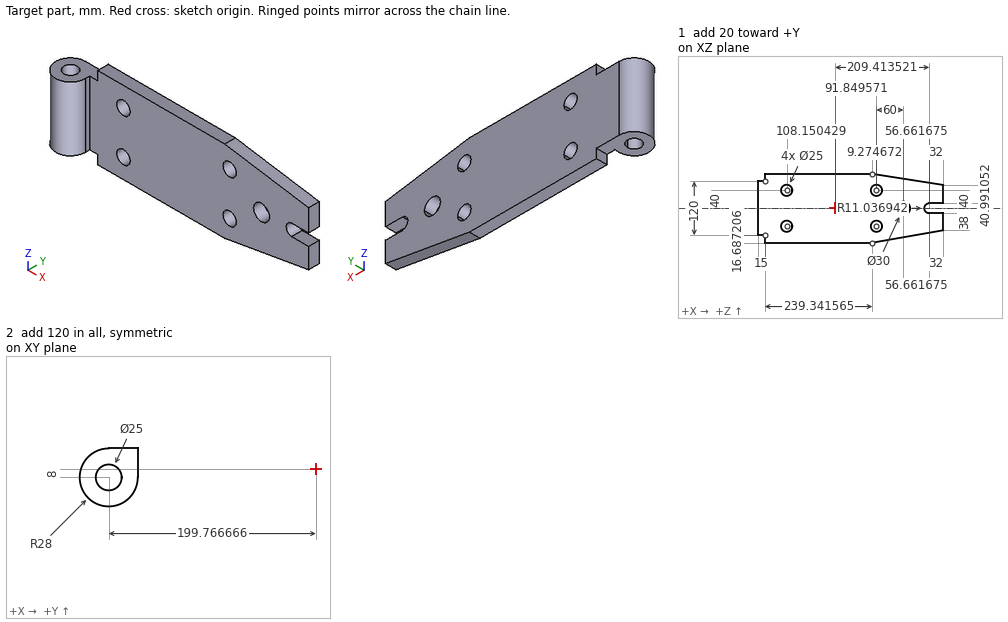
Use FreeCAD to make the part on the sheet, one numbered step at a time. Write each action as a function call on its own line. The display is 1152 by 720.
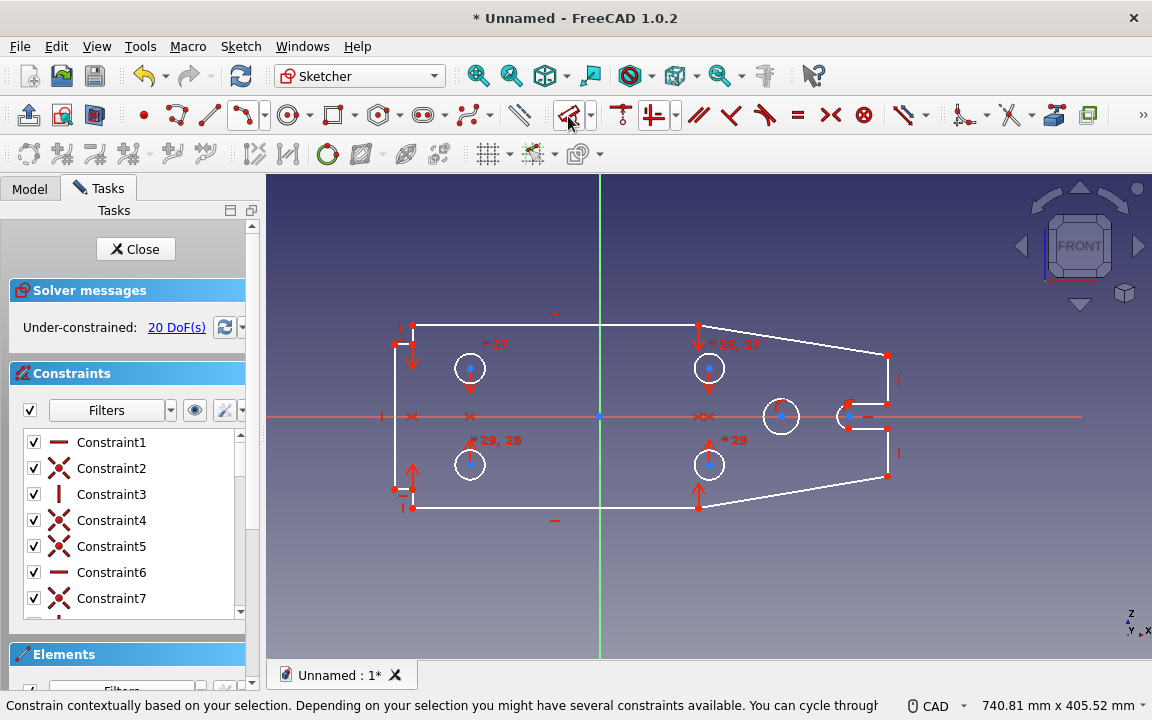
scroll(837, 417, up, 6)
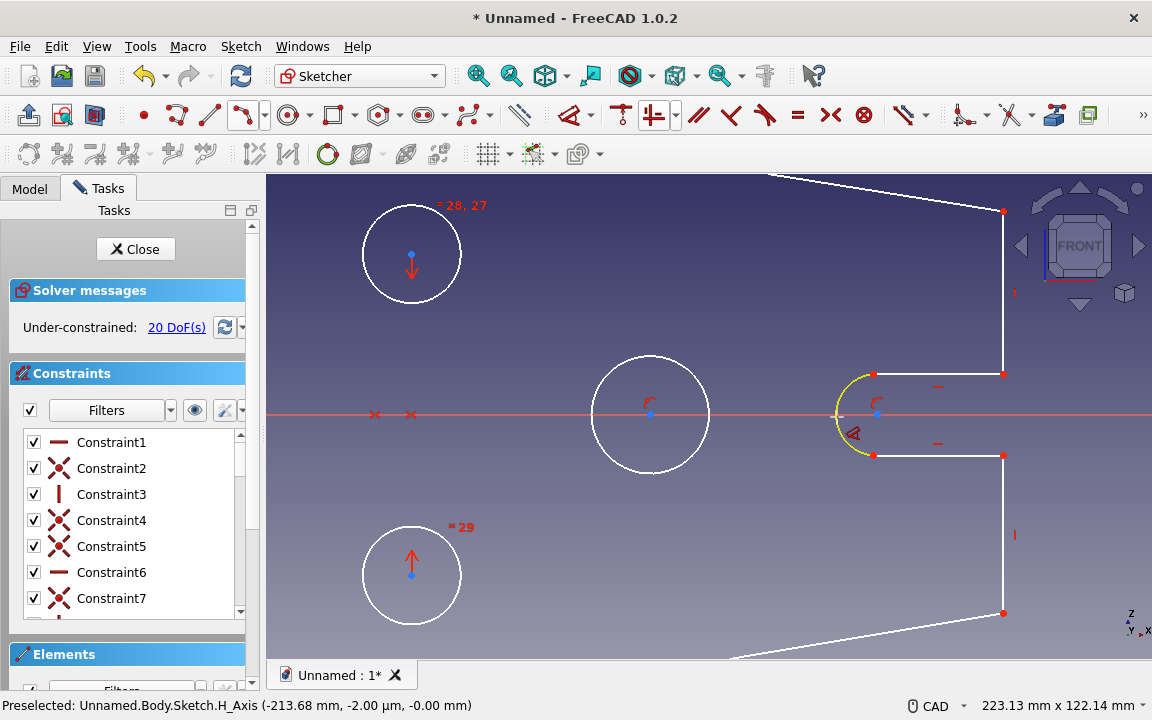
click(836, 415)
click(813, 380)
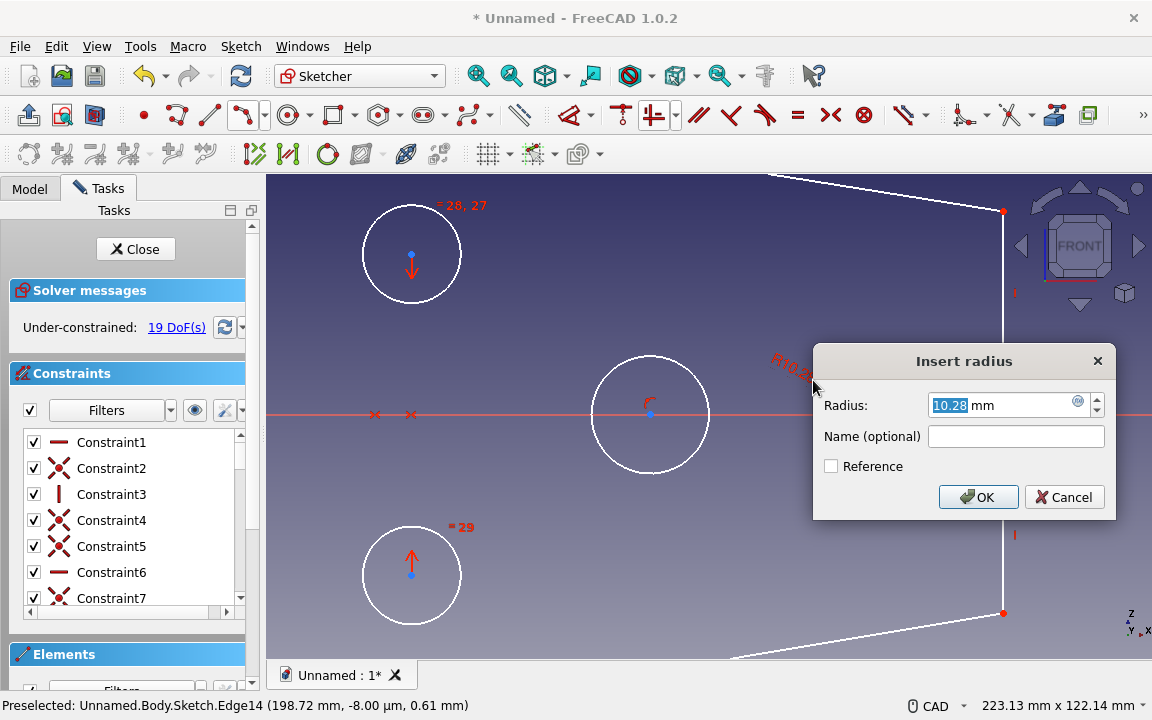
text(11.036942)
key(Return)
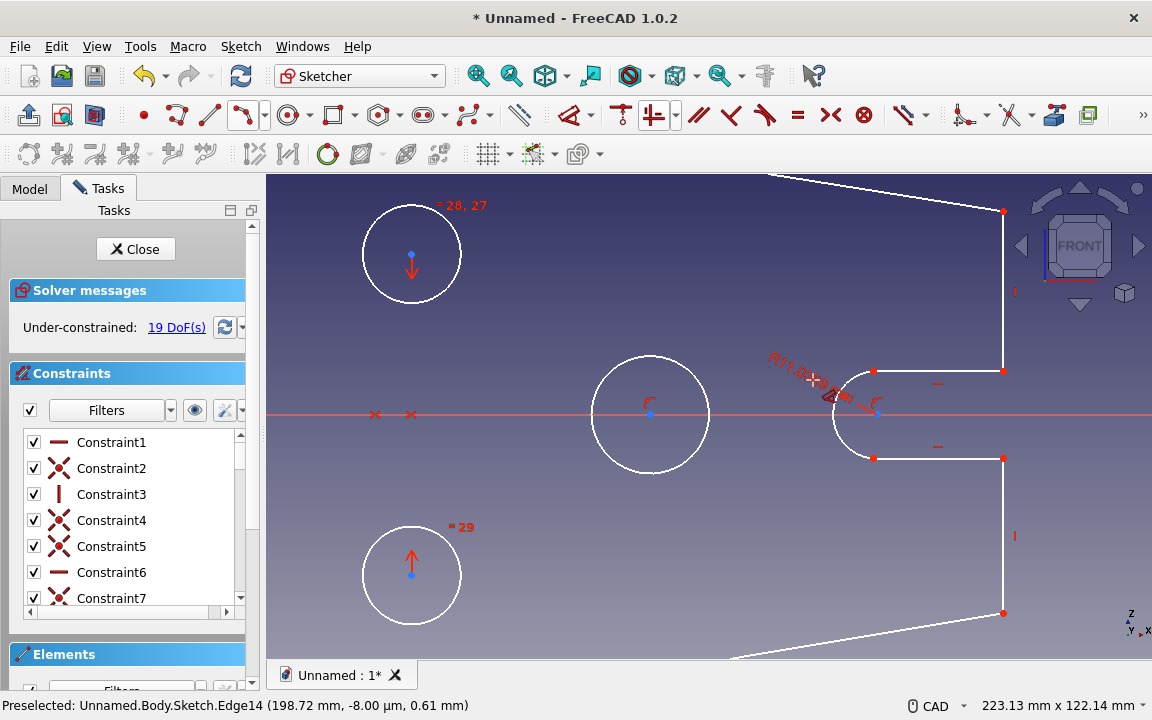
scroll(837, 417, down, 6)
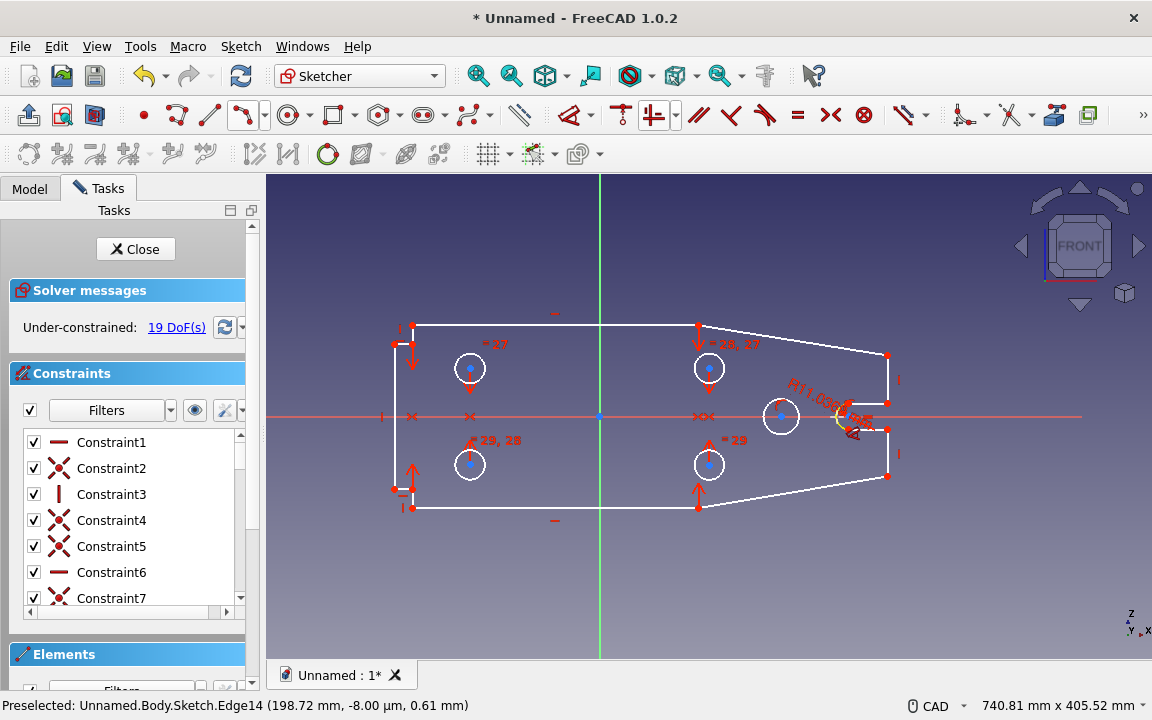
scroll(480, 358, up, 2)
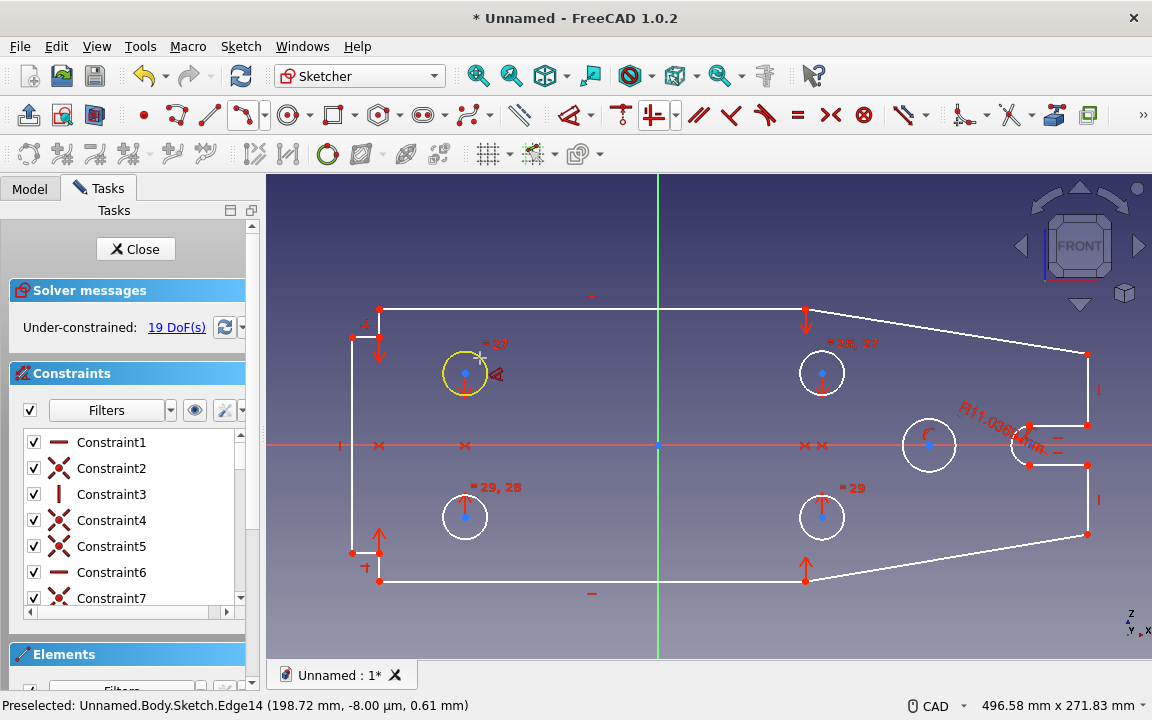
click(481, 358)
click(504, 336)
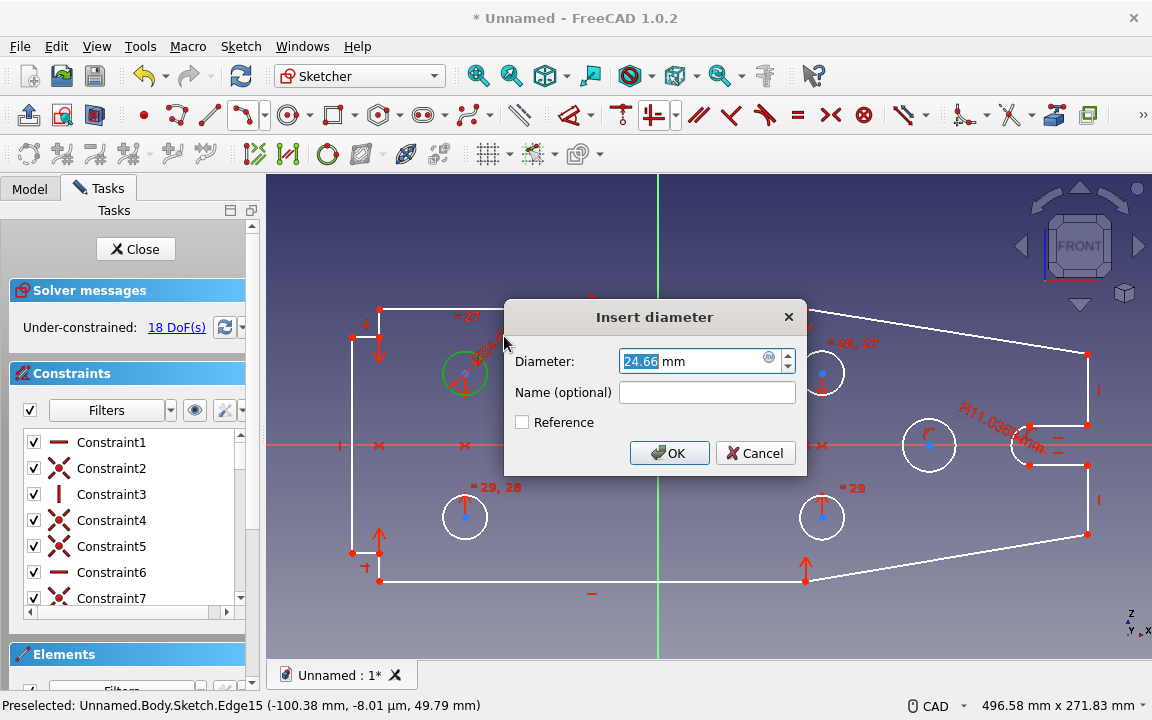
text(25)
key(Return)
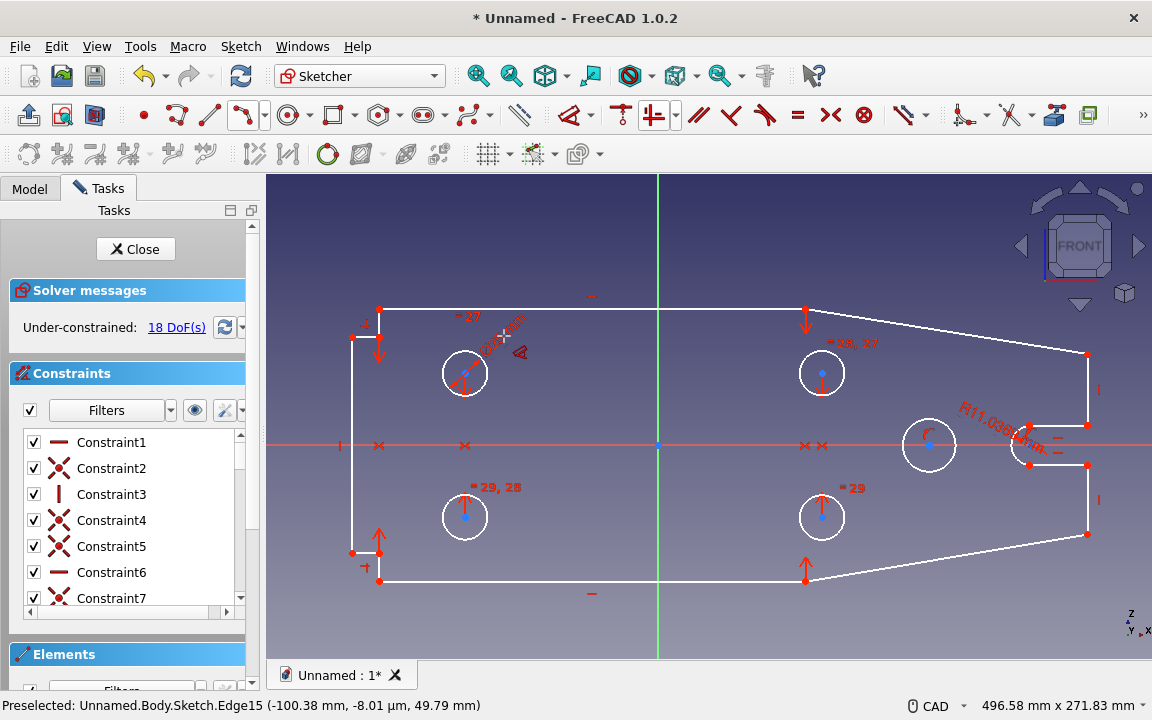
click(948, 427)
click(971, 405)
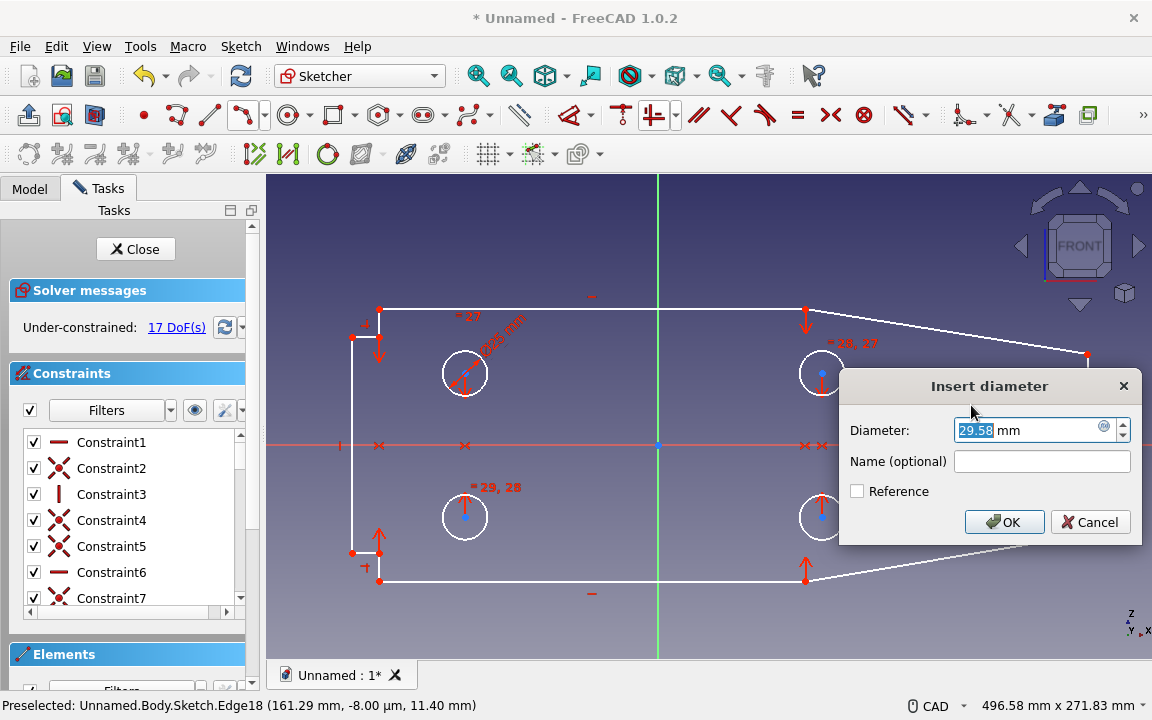
text(30)
key(Return)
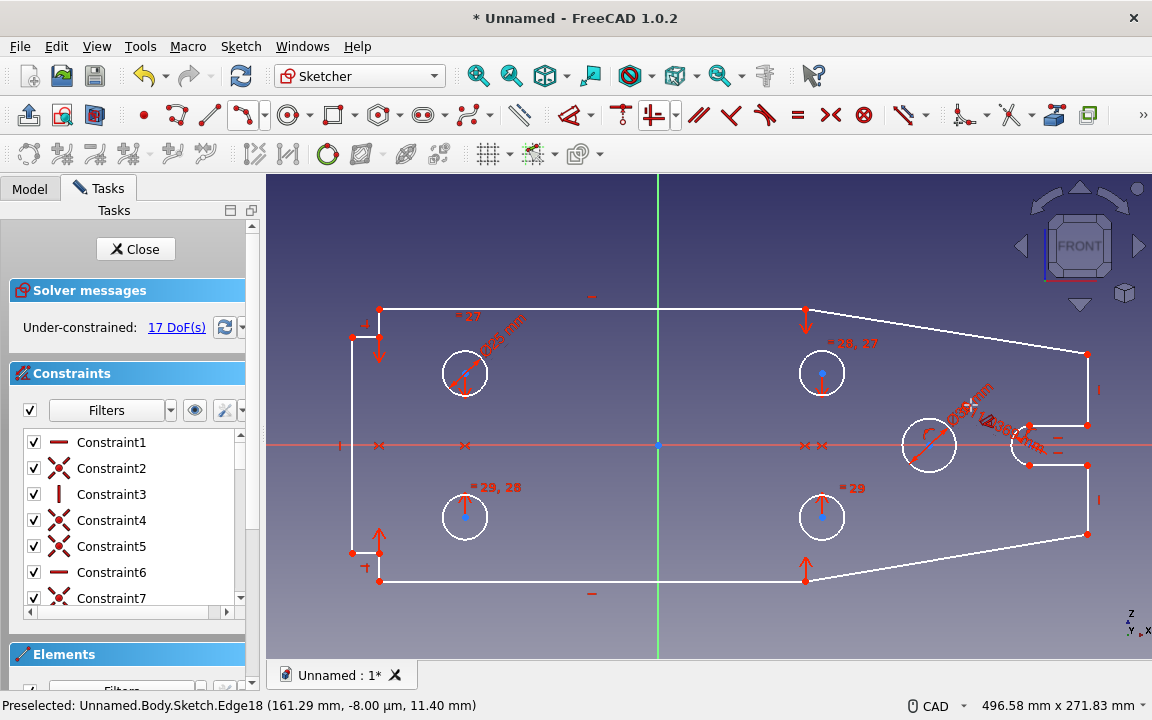
scroll(480, 358, down, 2)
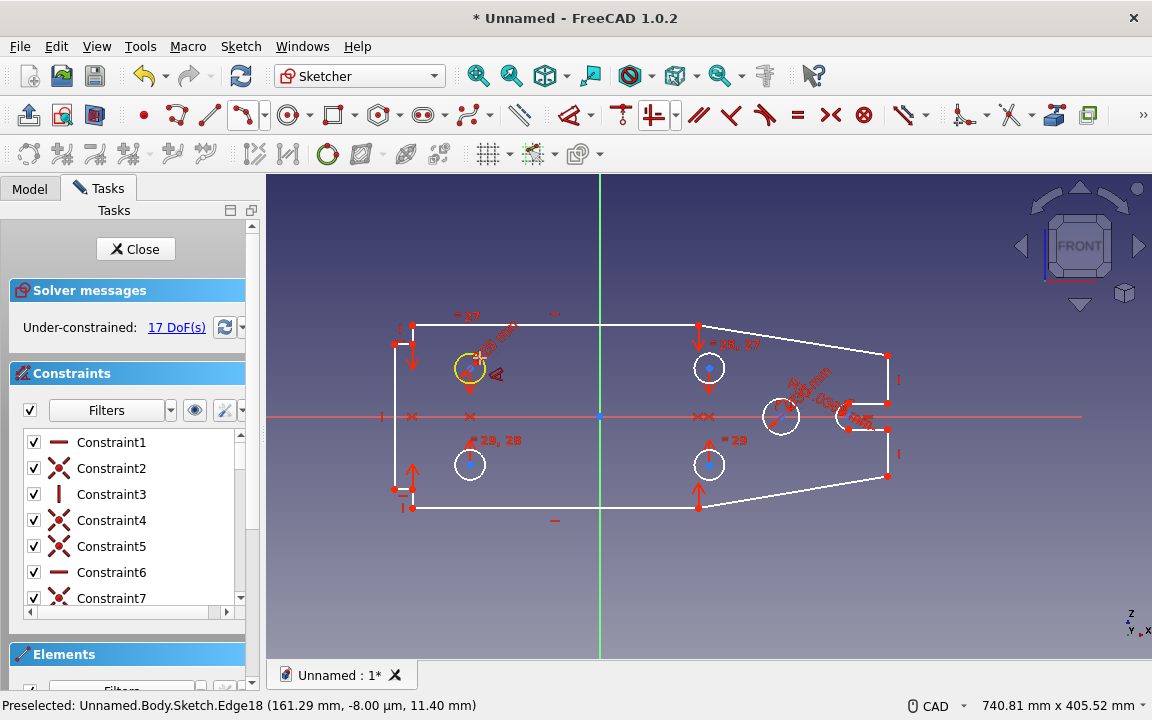
click(860, 430)
click(868, 464)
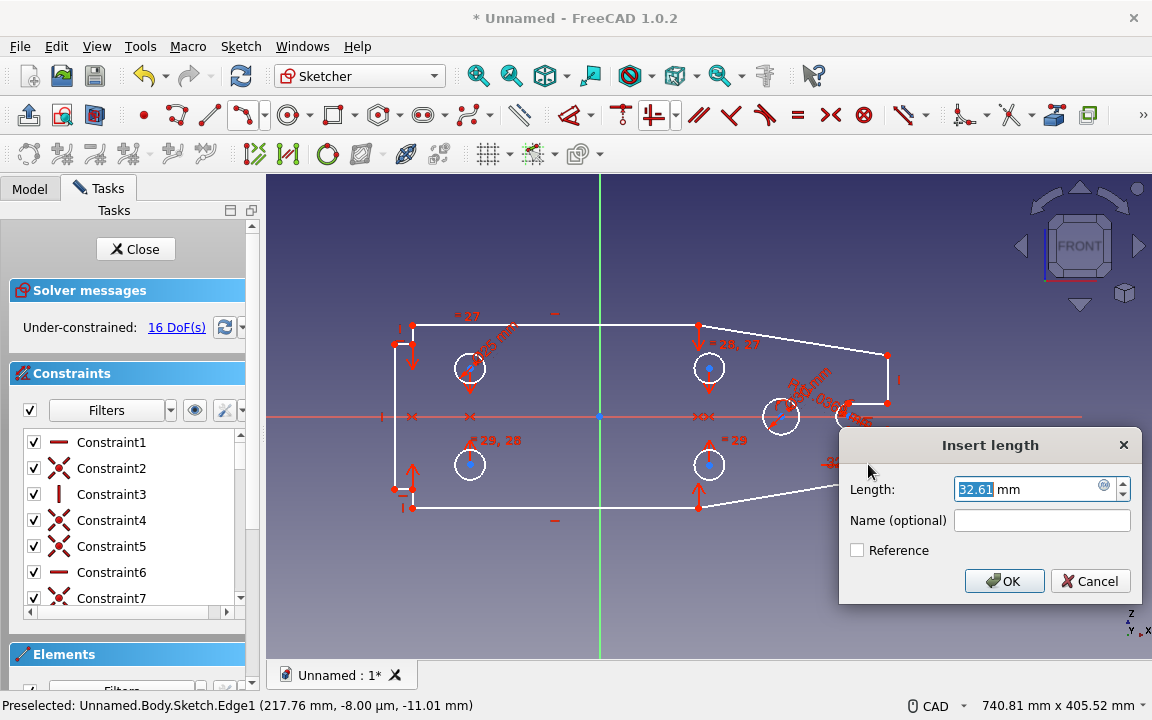
text(32)
key(Return)